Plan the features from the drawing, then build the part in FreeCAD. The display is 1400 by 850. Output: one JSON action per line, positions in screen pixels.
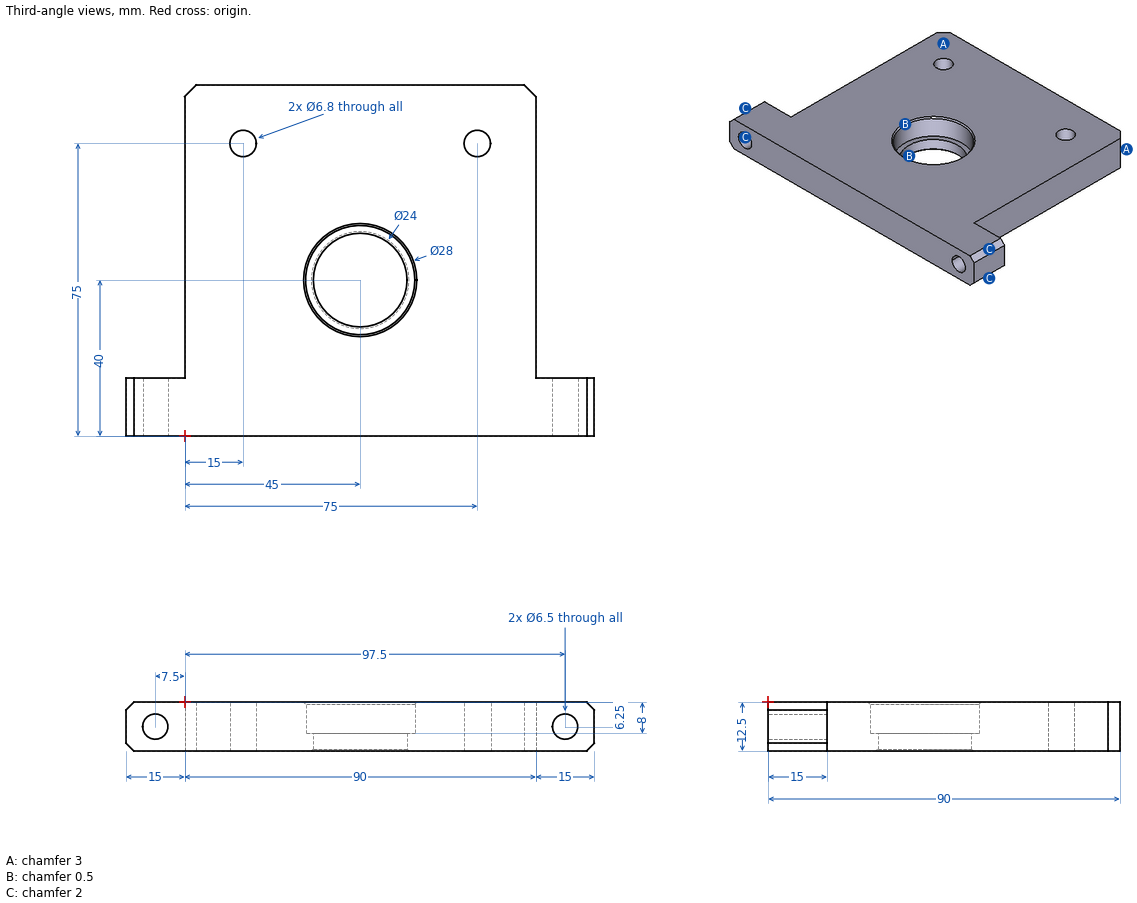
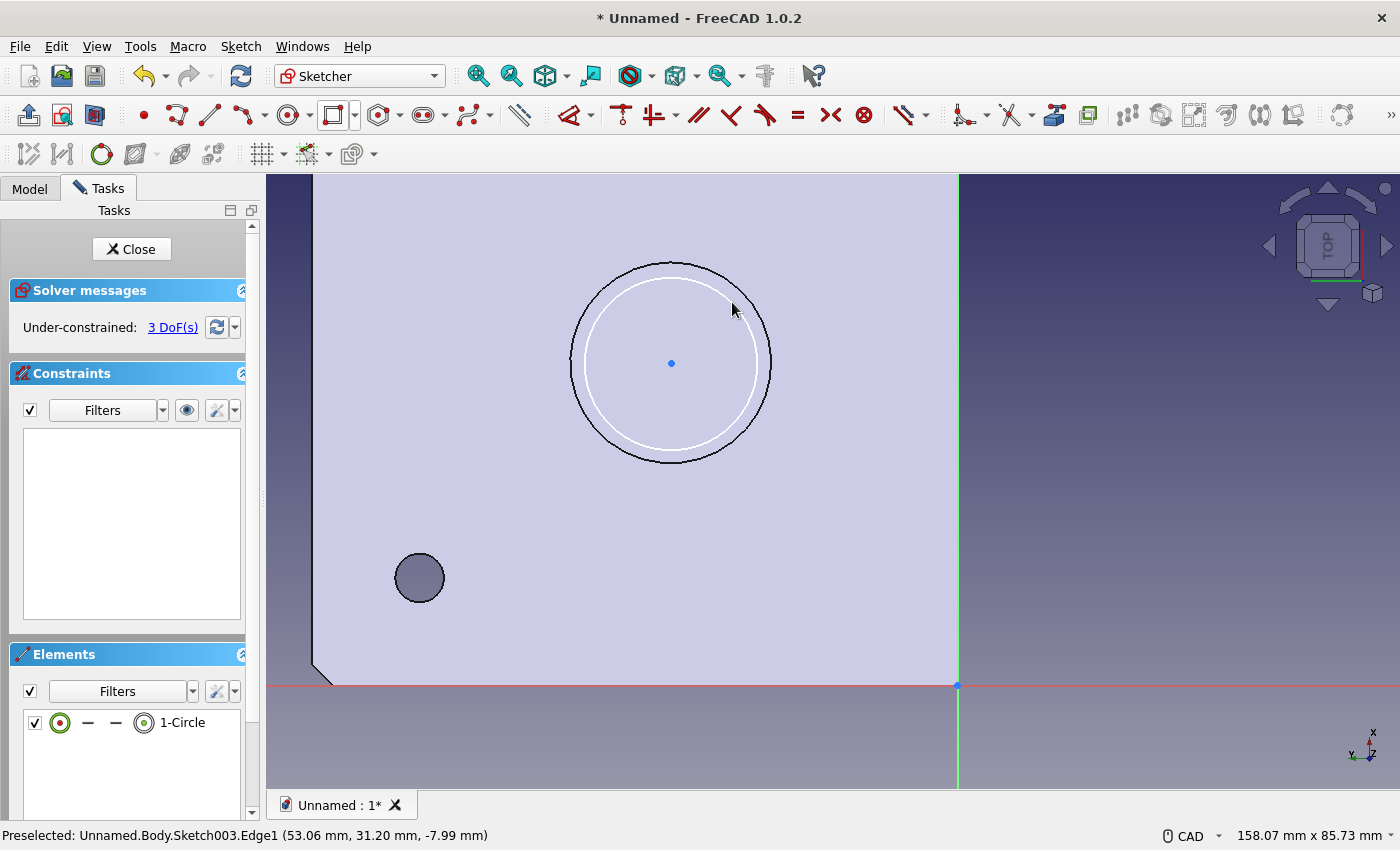
{"action": "left_click", "coordinate": [568, 116]}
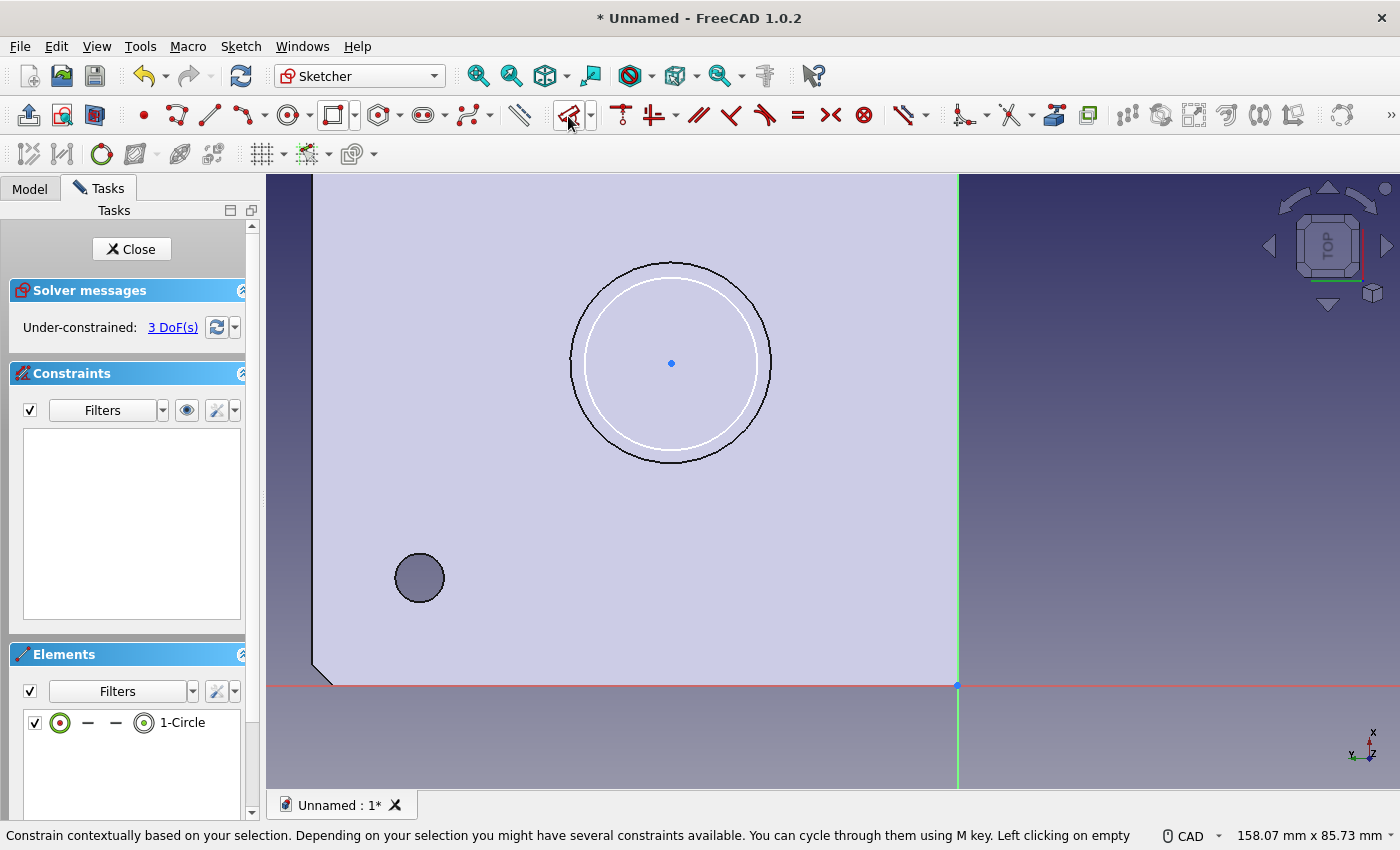
{"action": "left_click", "coordinate": [732, 303]}
{"action": "left_click", "coordinate": [755, 280]}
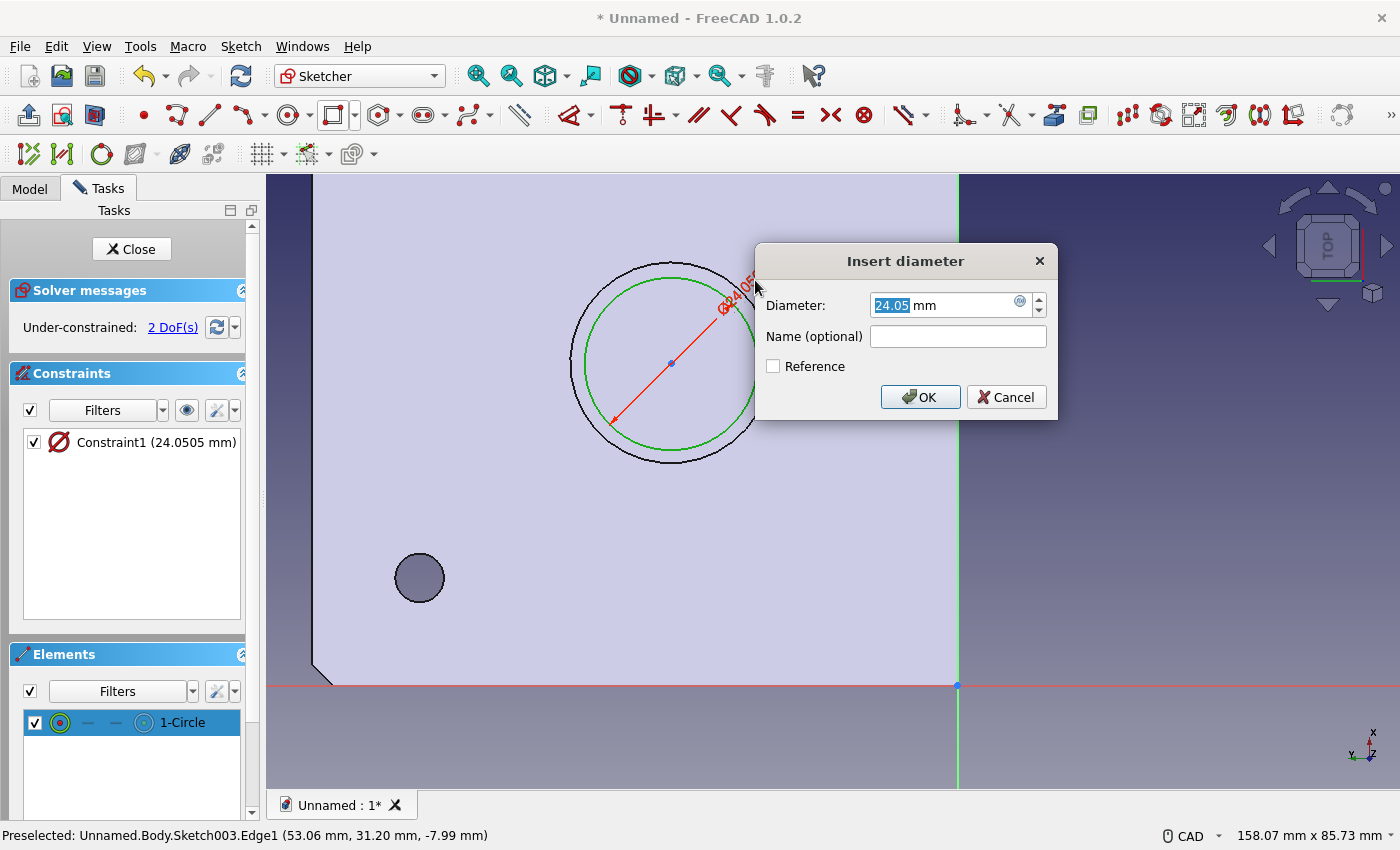
{"action": "type", "text": "24"}
{"action": "key", "text": "Return"}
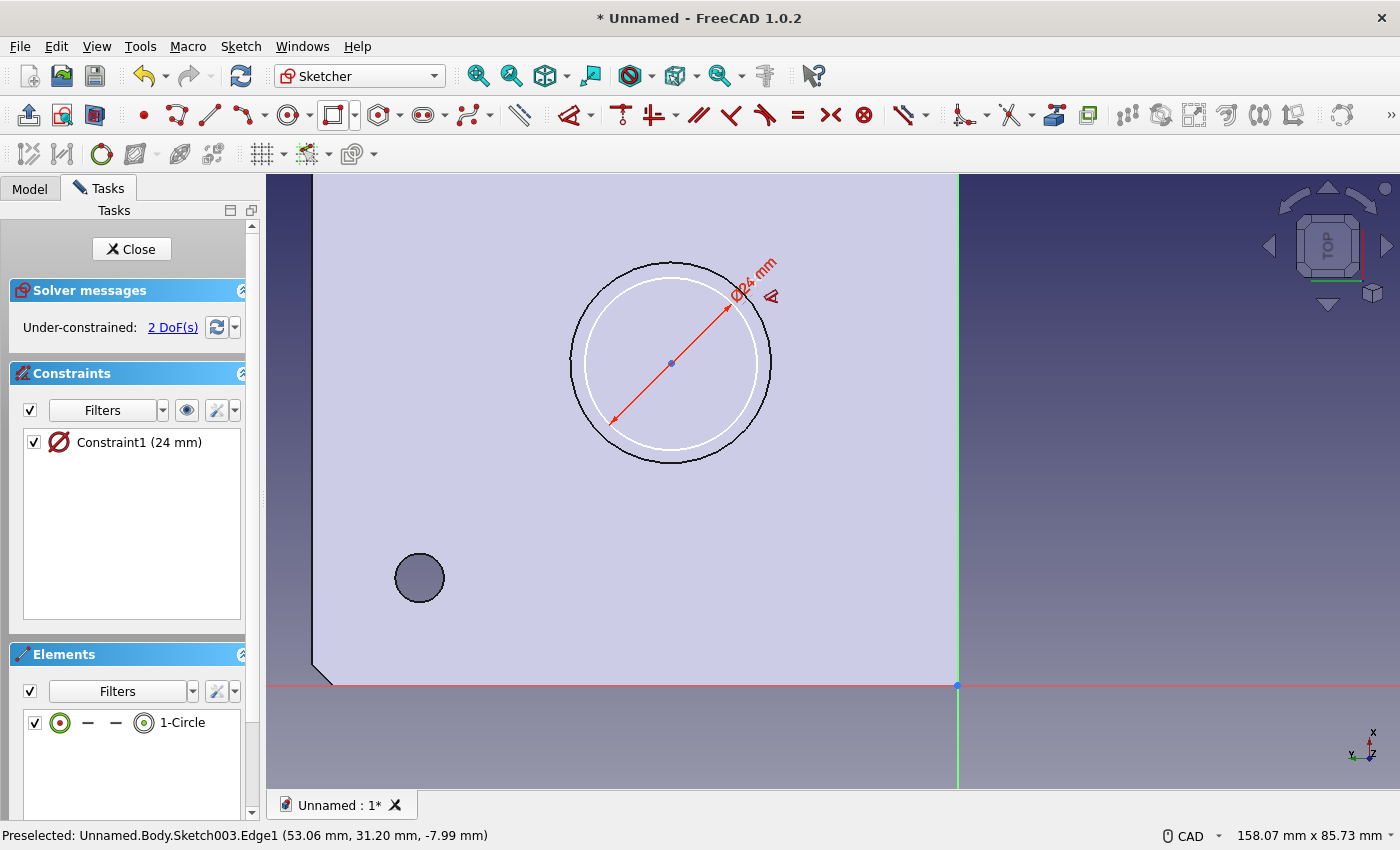
{"action": "left_click", "coordinate": [671, 364]}
{"action": "left_click", "coordinate": [814, 720]}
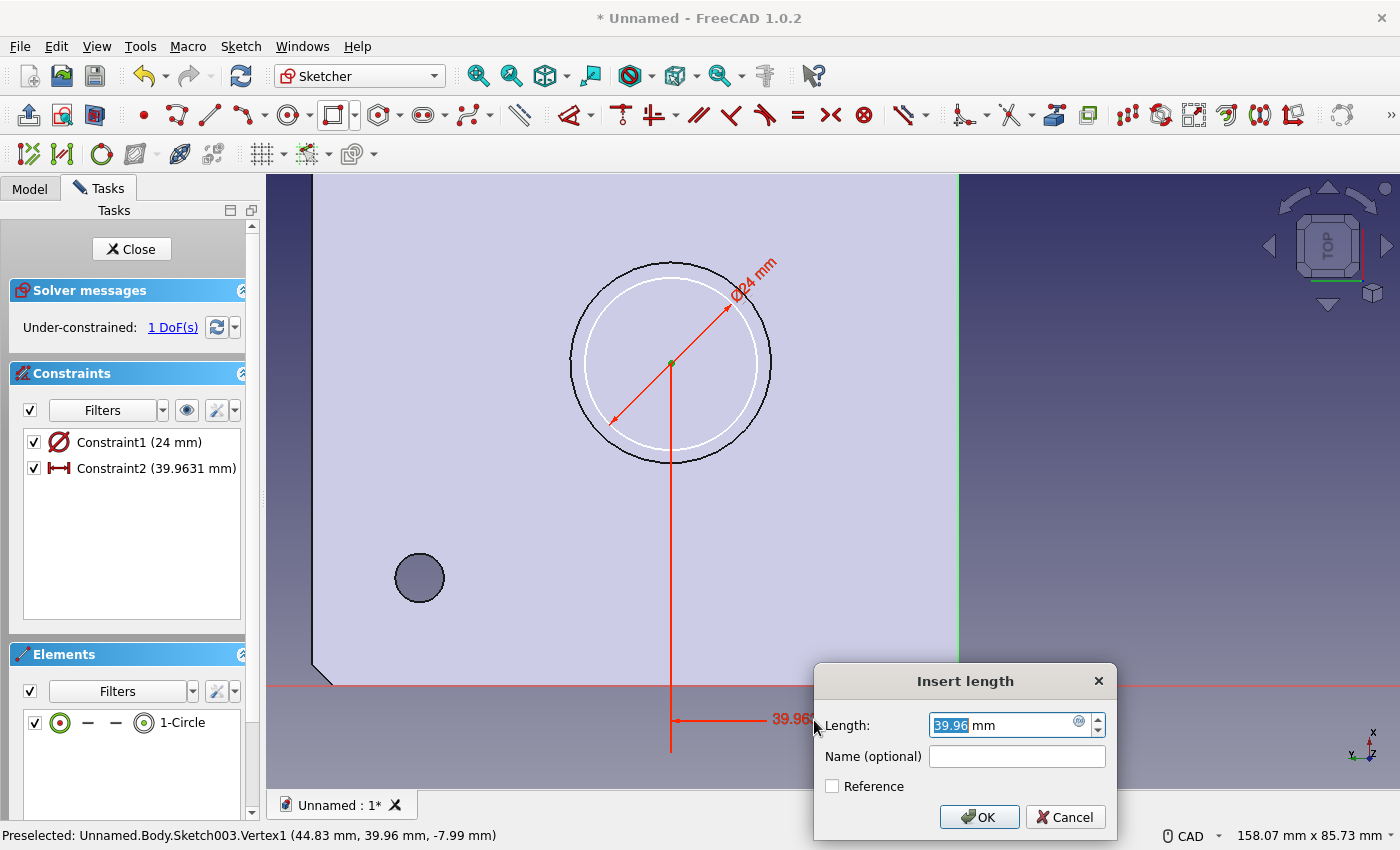
{"action": "type", "text": "40"}
{"action": "key", "text": "Return"}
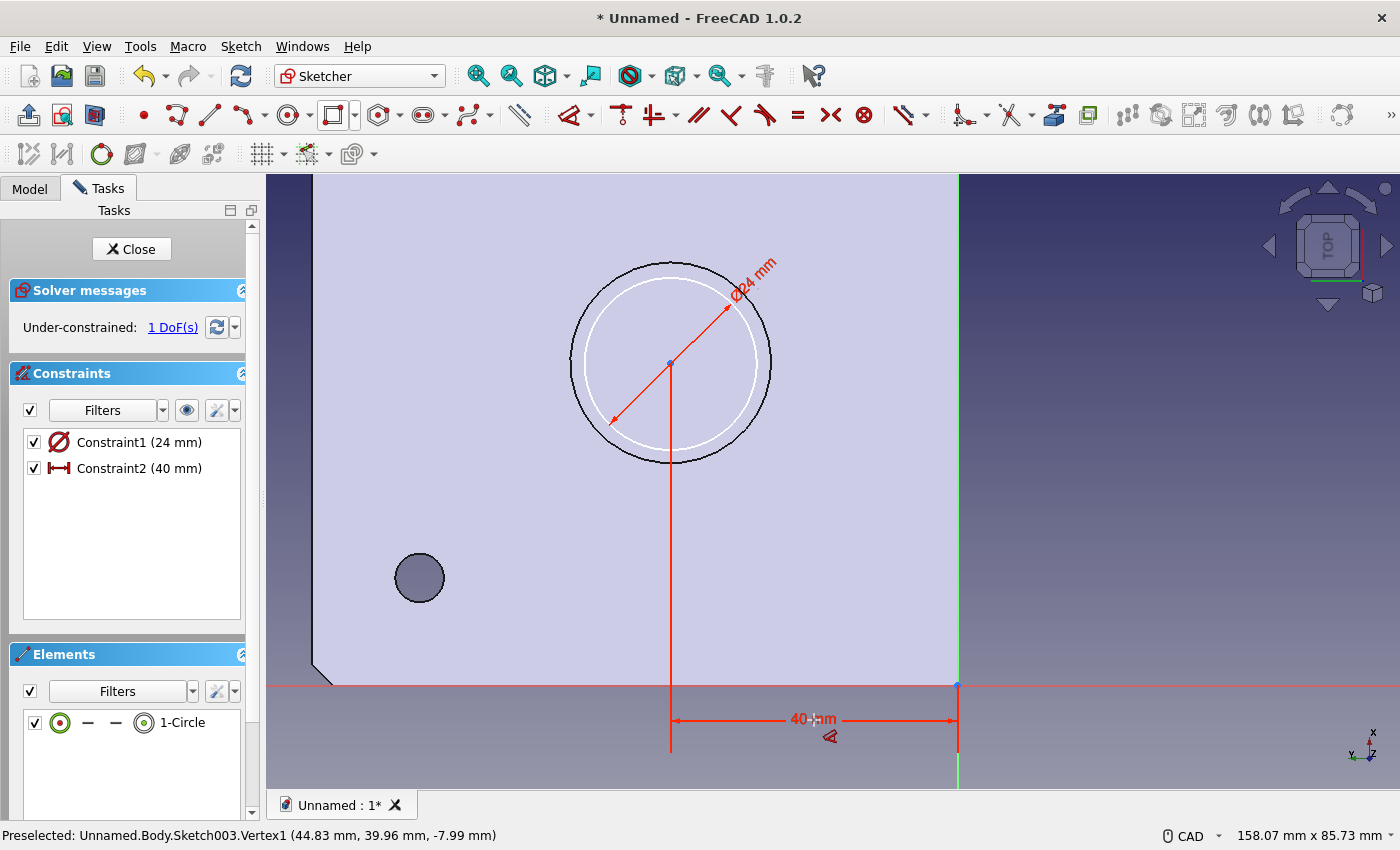
{"action": "left_click", "coordinate": [671, 364]}
{"action": "left_click", "coordinate": [992, 525]}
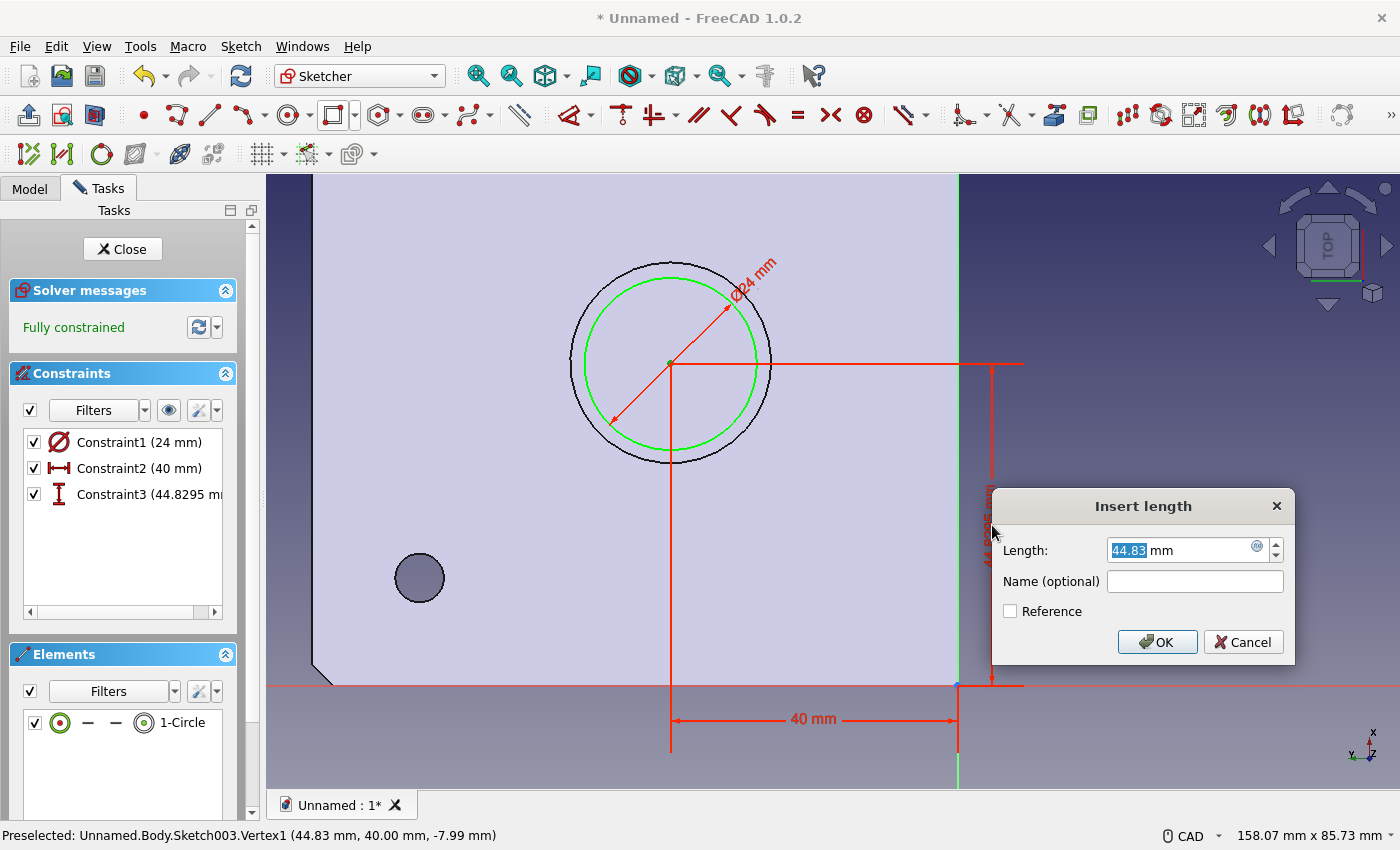
{"action": "type", "text": "45"}
{"action": "key", "text": "Return"}
{"action": "key", "text": "Escape"}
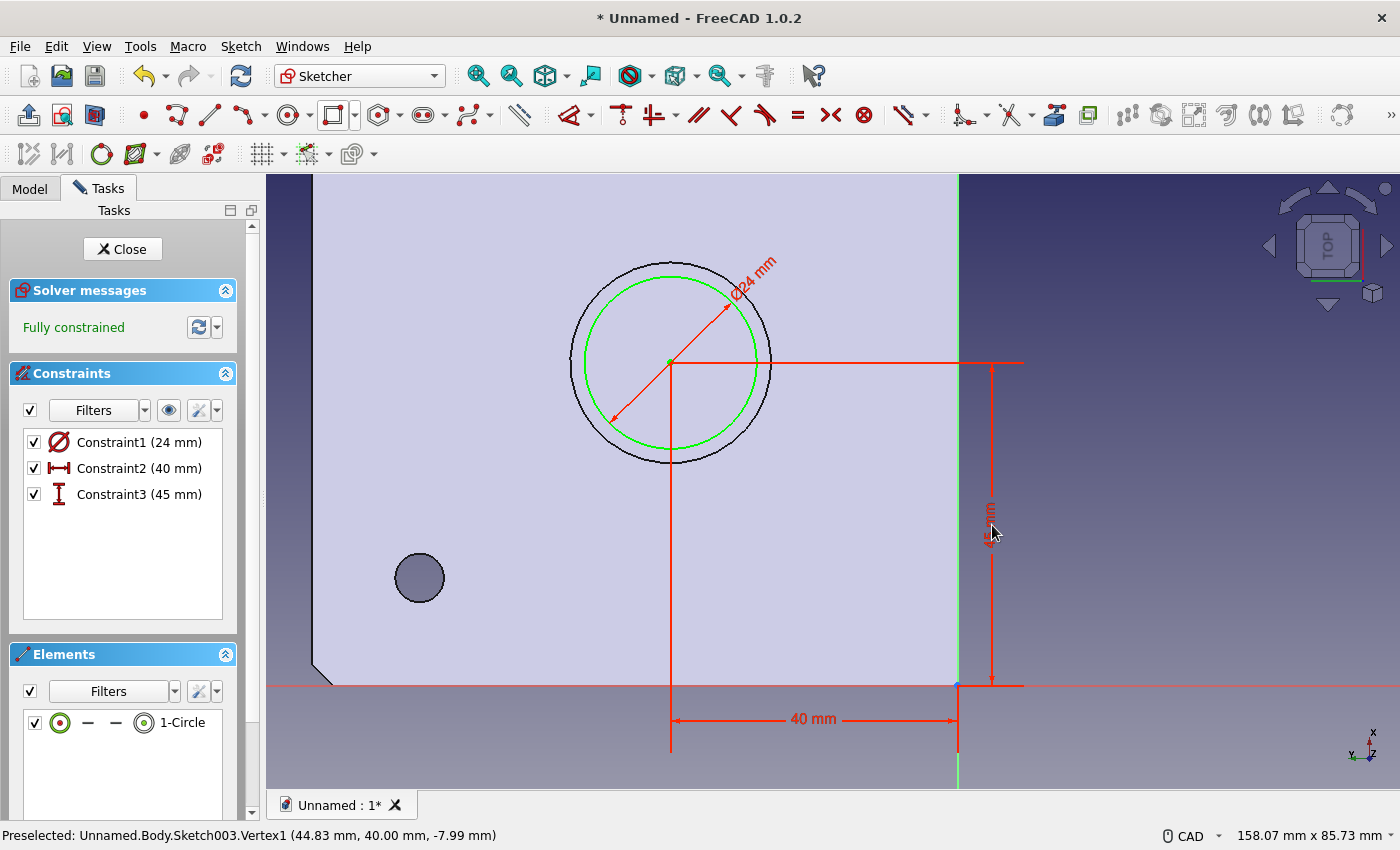
{"action": "left_click", "coordinate": [123, 249]}